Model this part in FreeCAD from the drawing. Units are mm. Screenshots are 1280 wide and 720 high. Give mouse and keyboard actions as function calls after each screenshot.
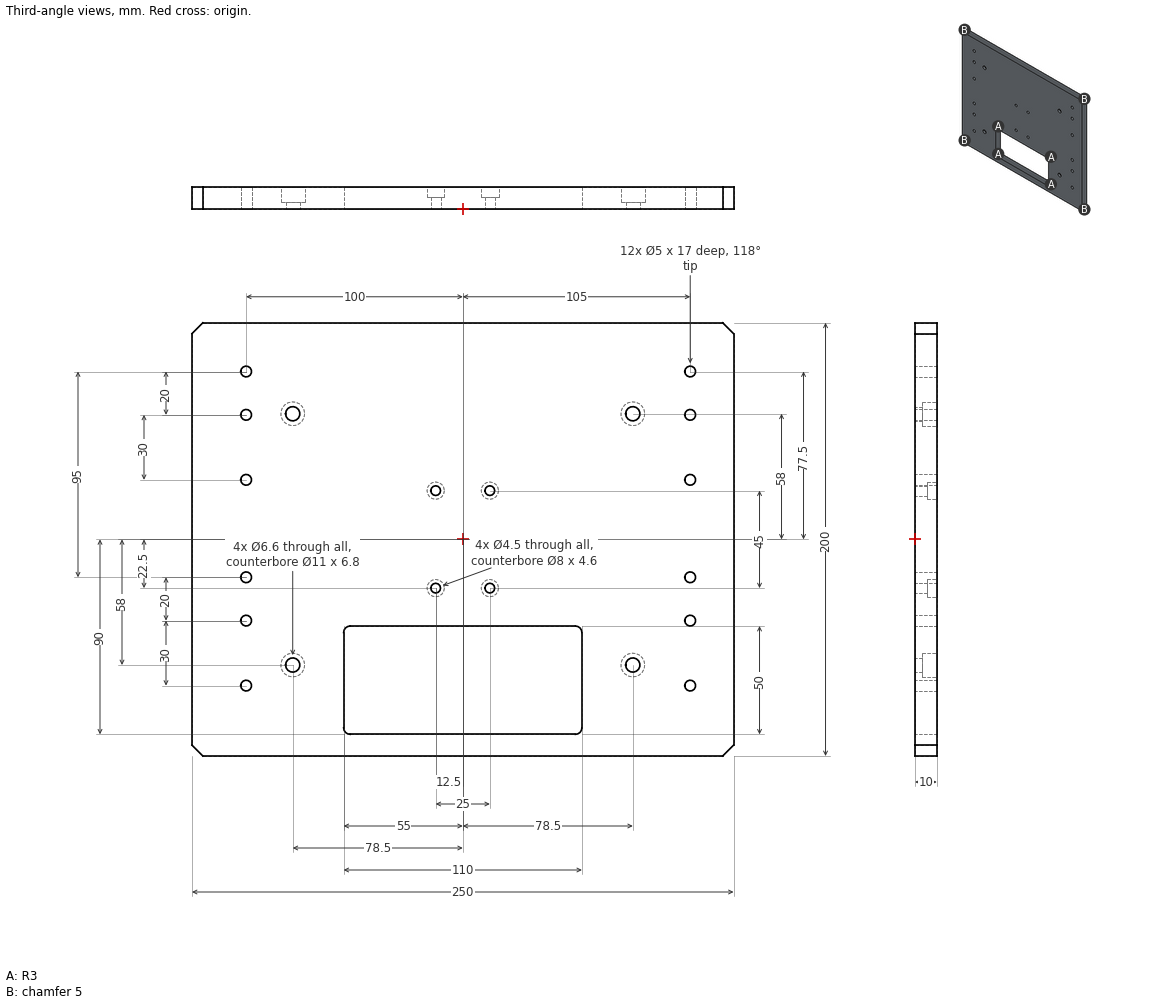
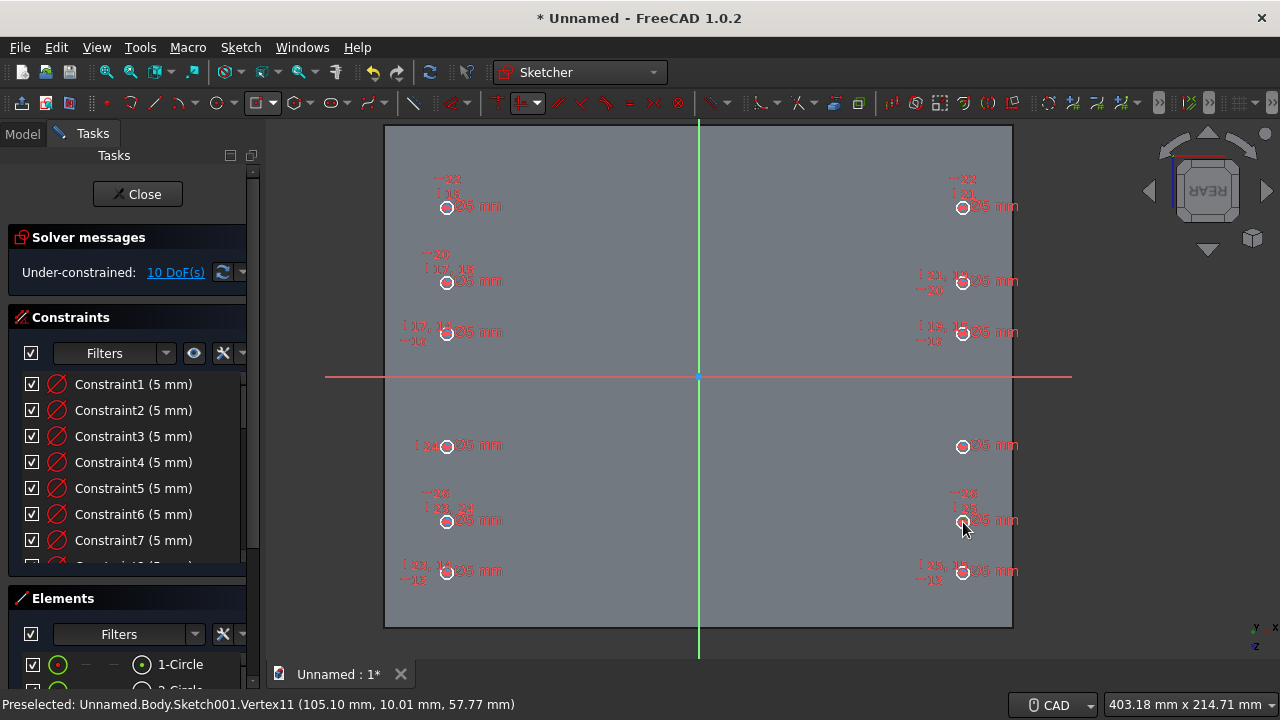
click(963, 447)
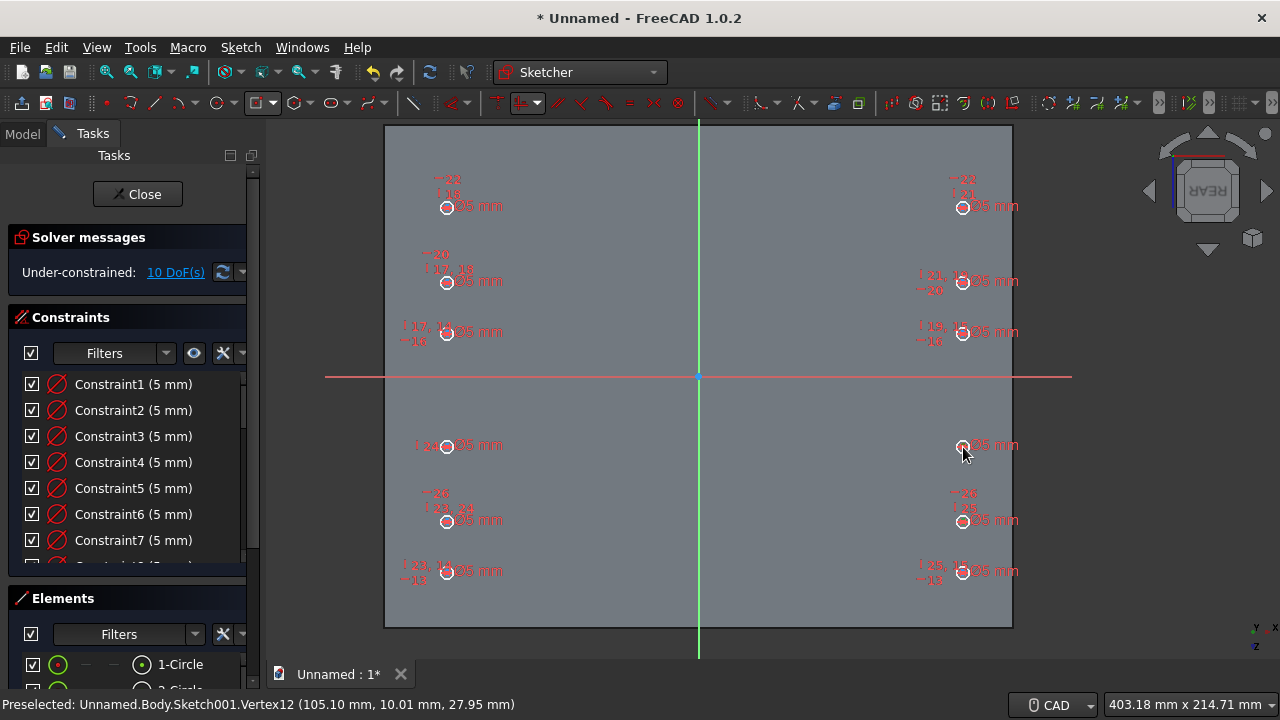
click(540, 104)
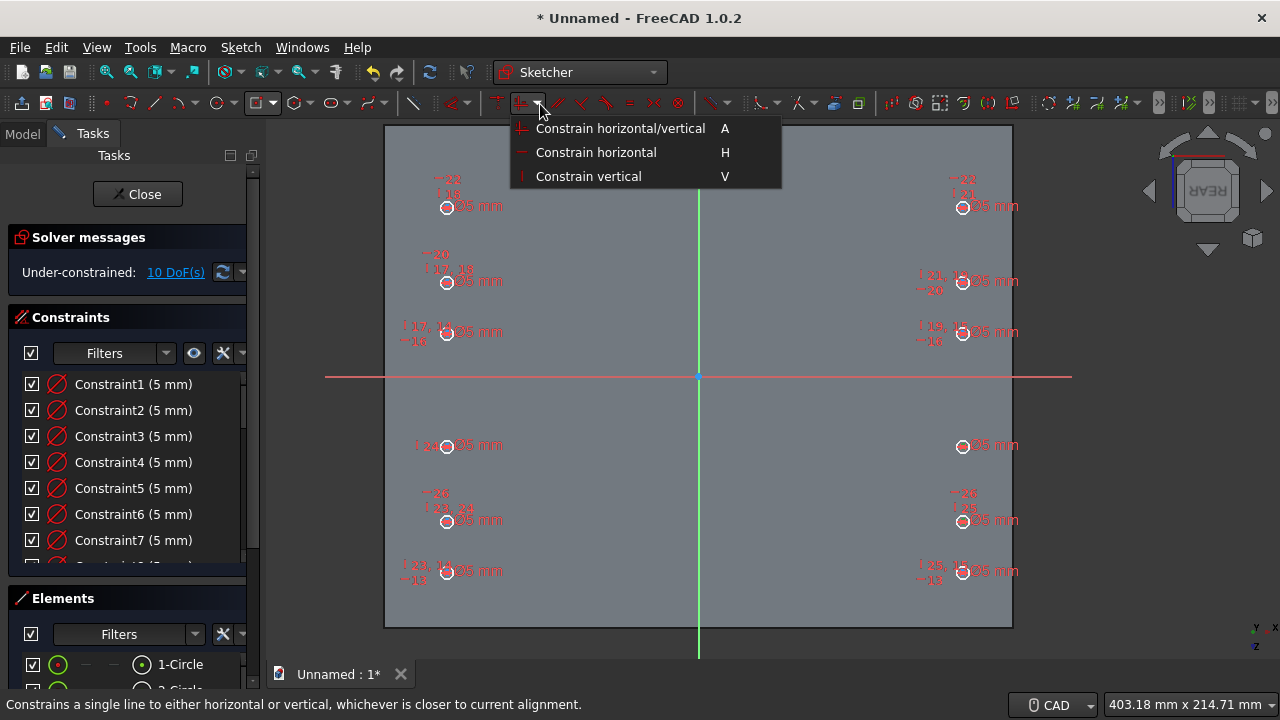
click(646, 176)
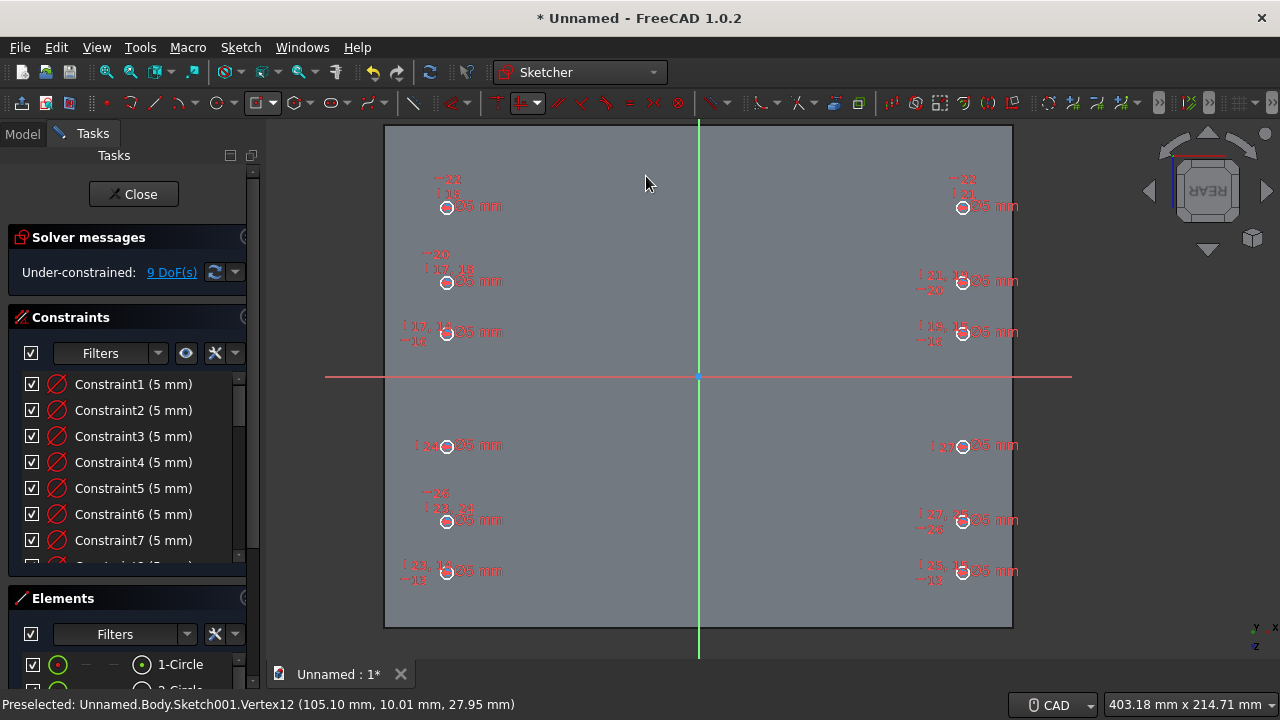
click(447, 447)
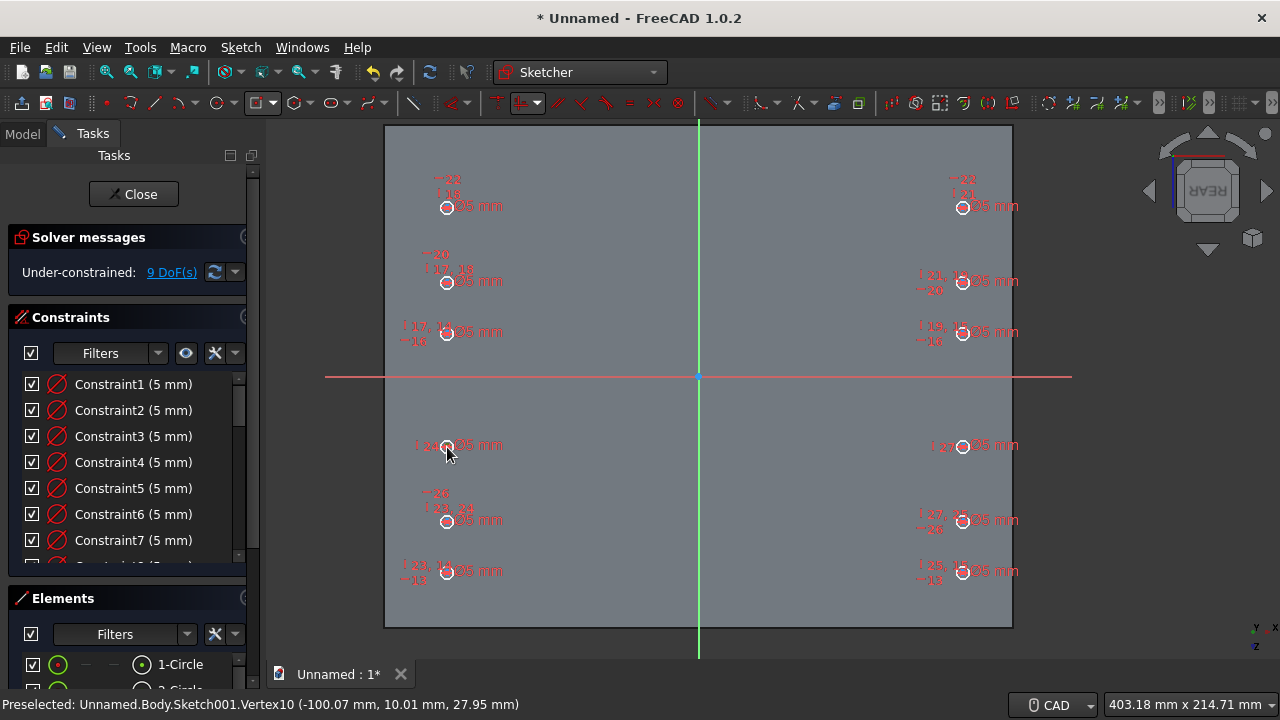
click(963, 447)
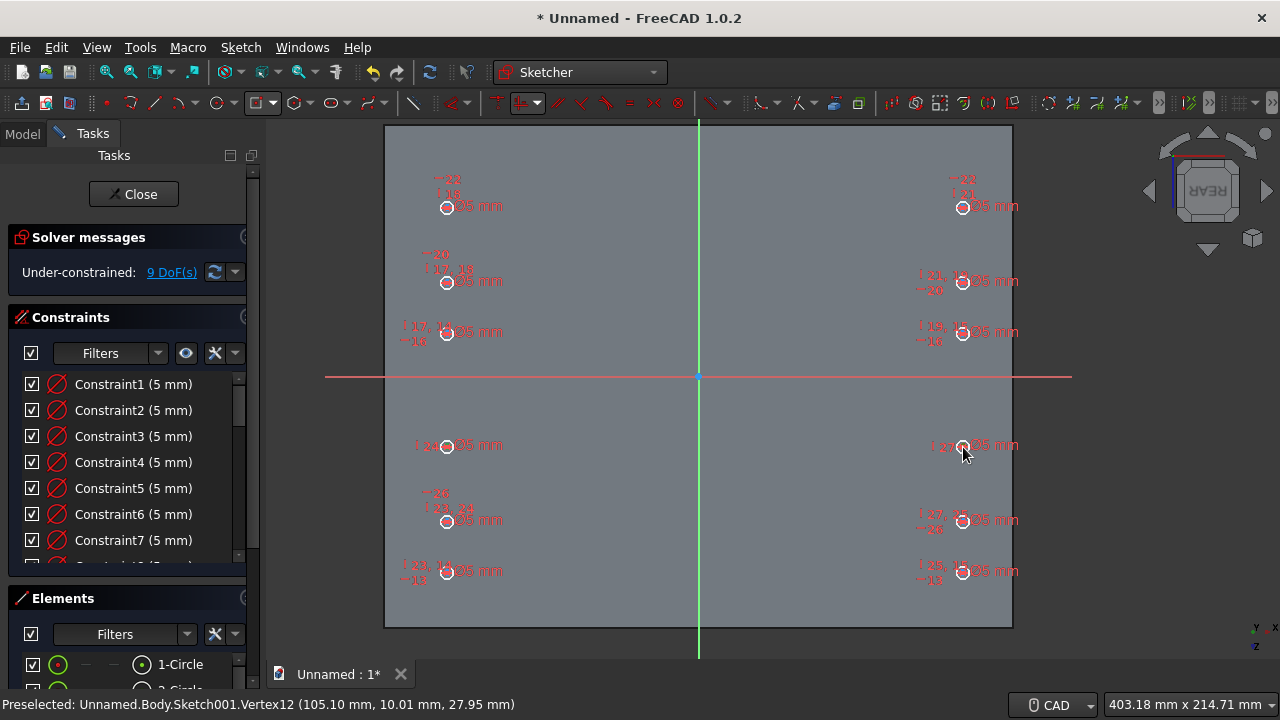
key(h)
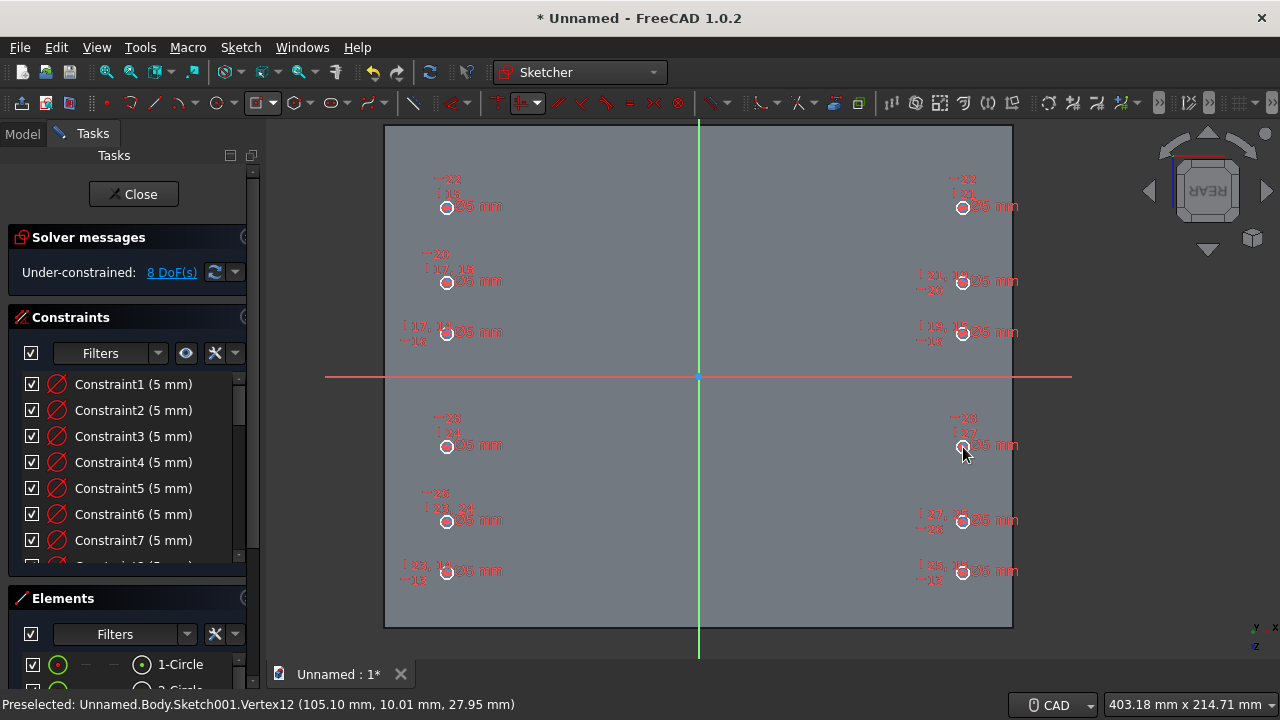
click(963, 573)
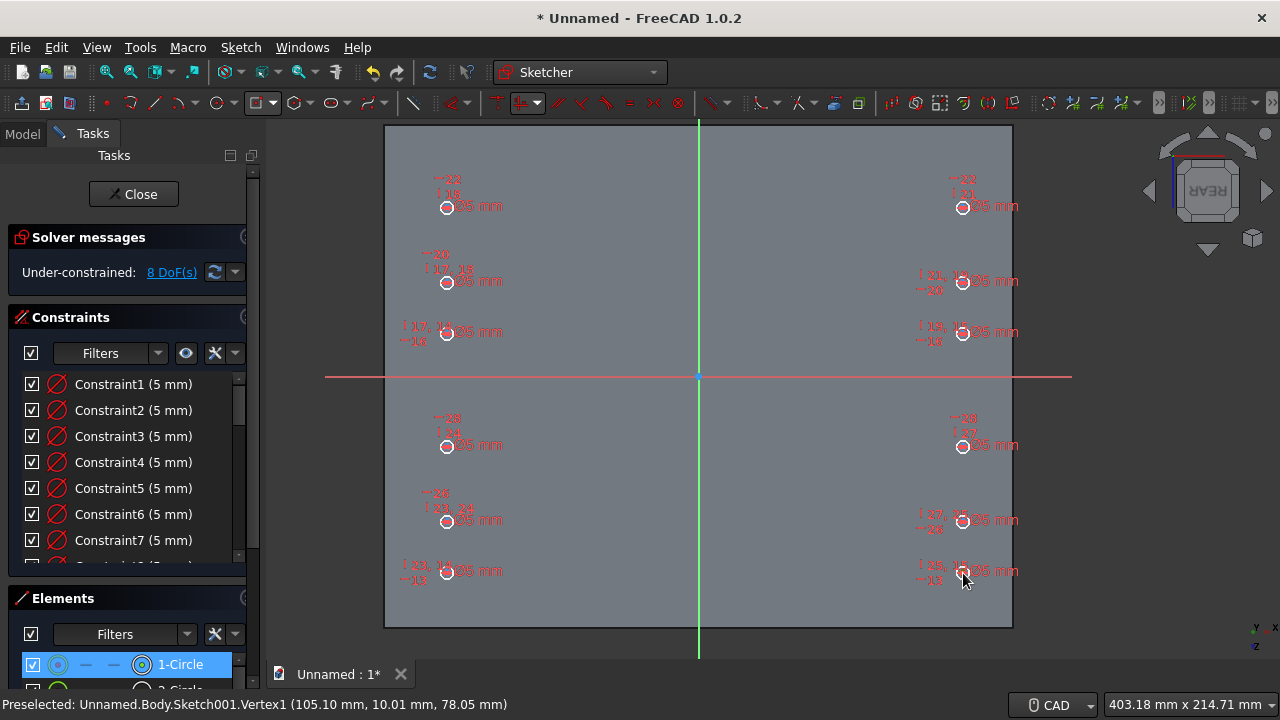
click(470, 104)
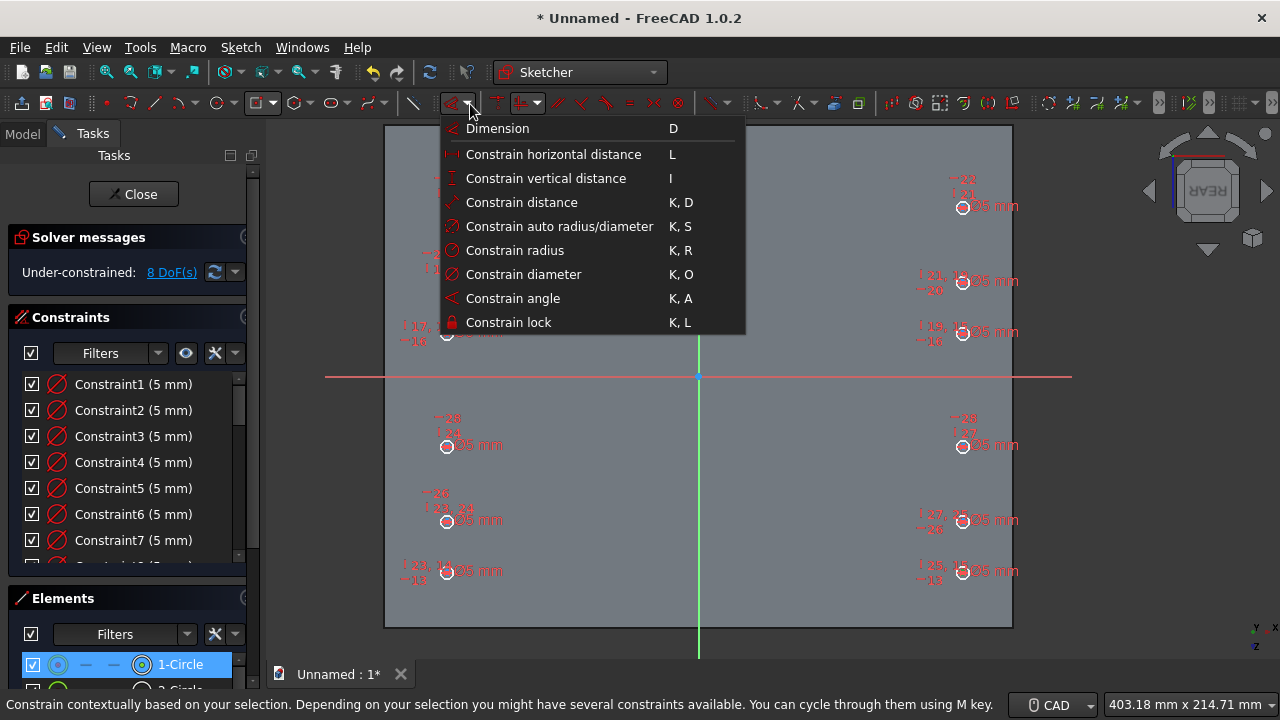
click(593, 154)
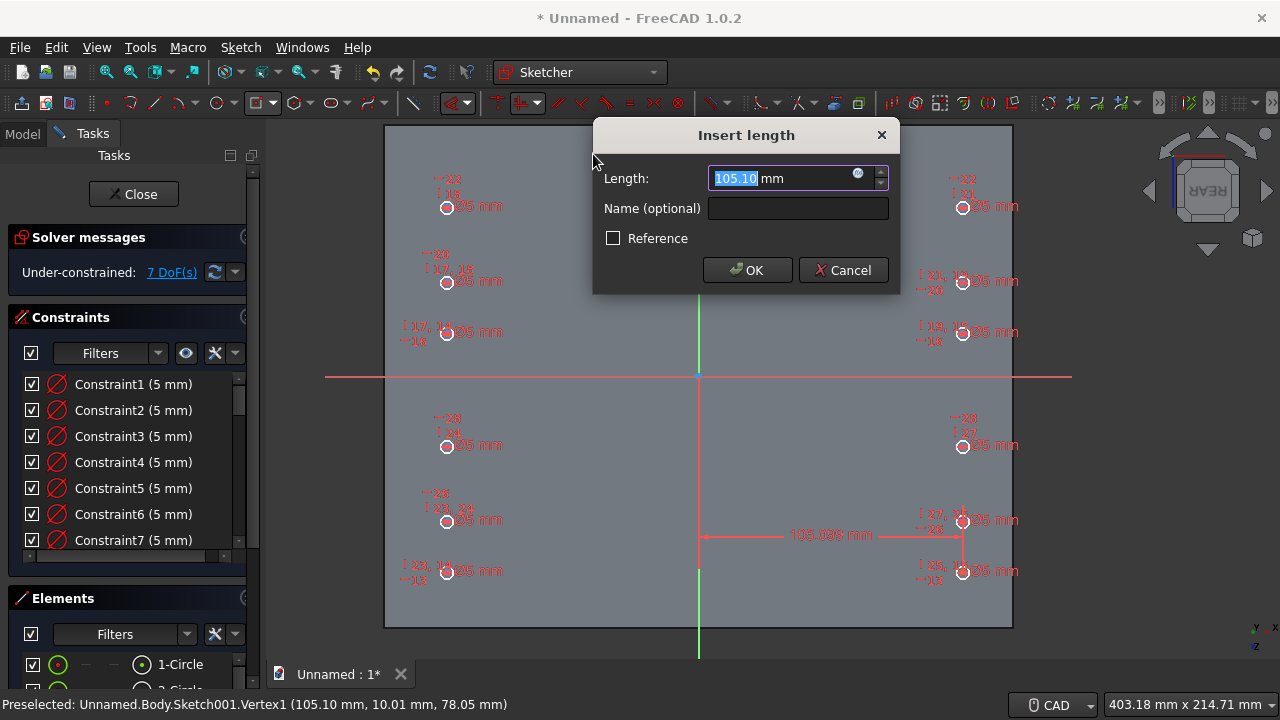
text(105)
key(Return)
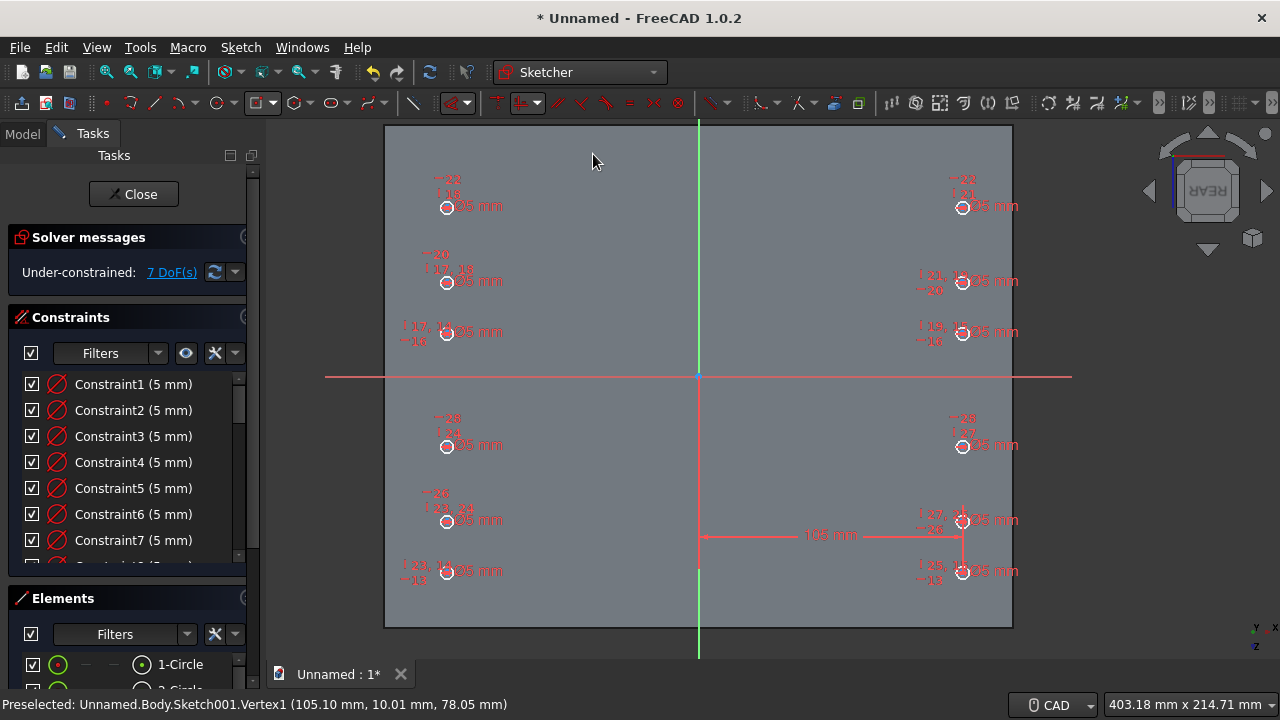
click(447, 573)